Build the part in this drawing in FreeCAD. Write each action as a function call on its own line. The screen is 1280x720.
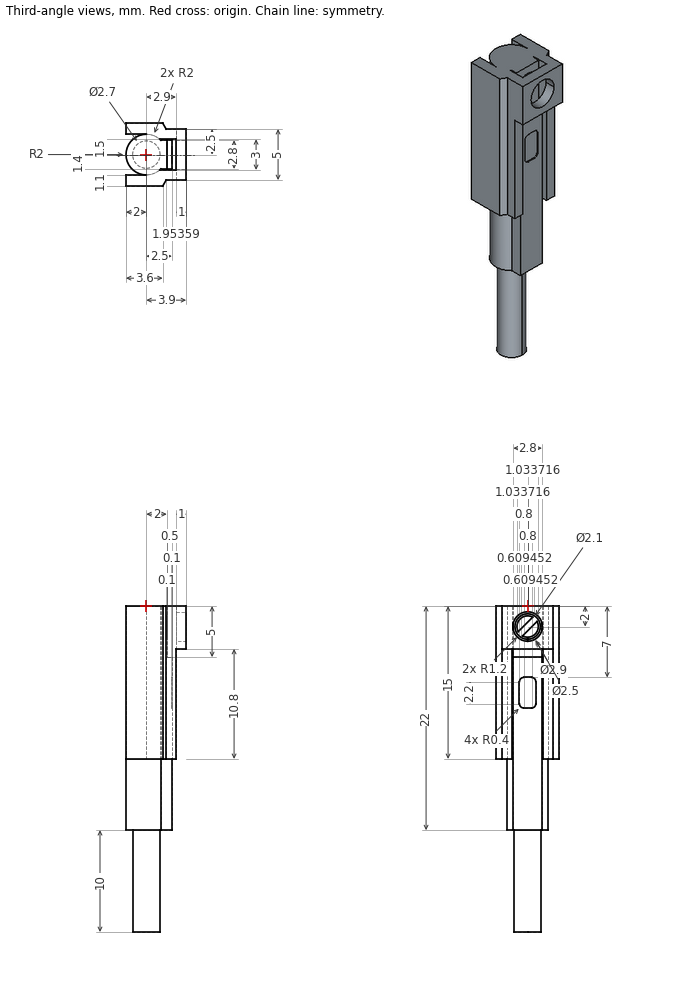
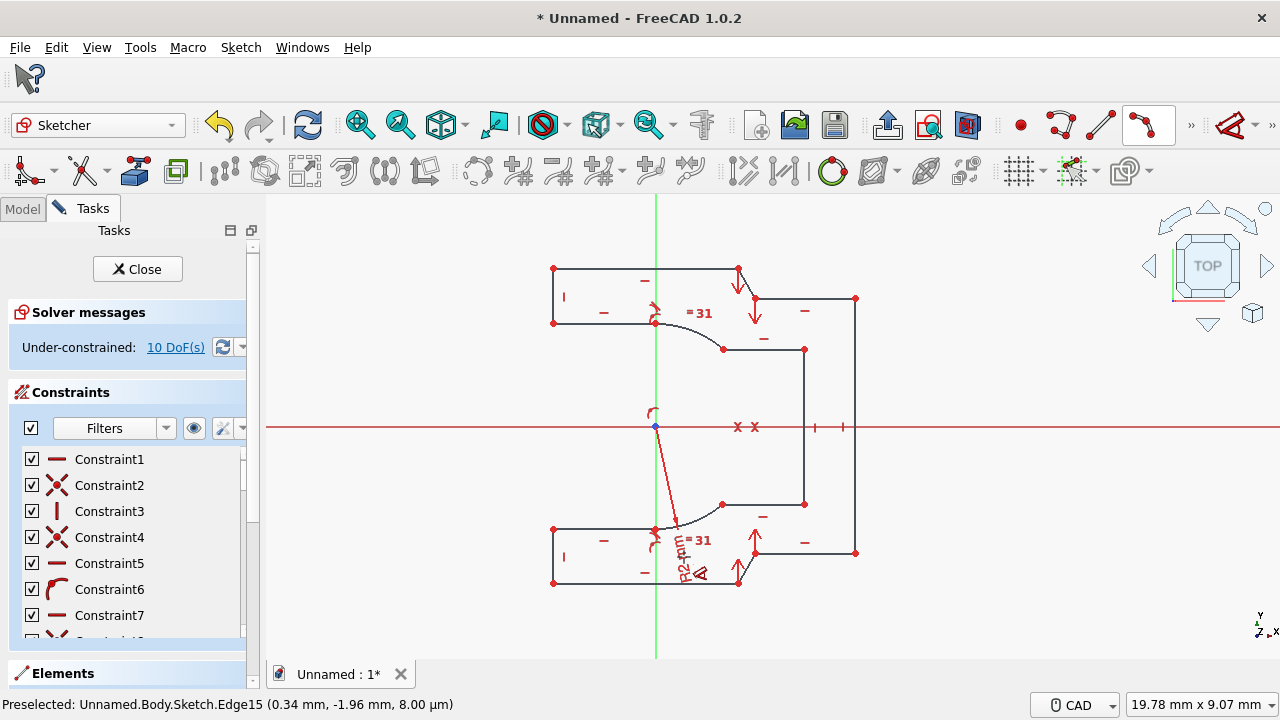
click(804, 396)
click(838, 392)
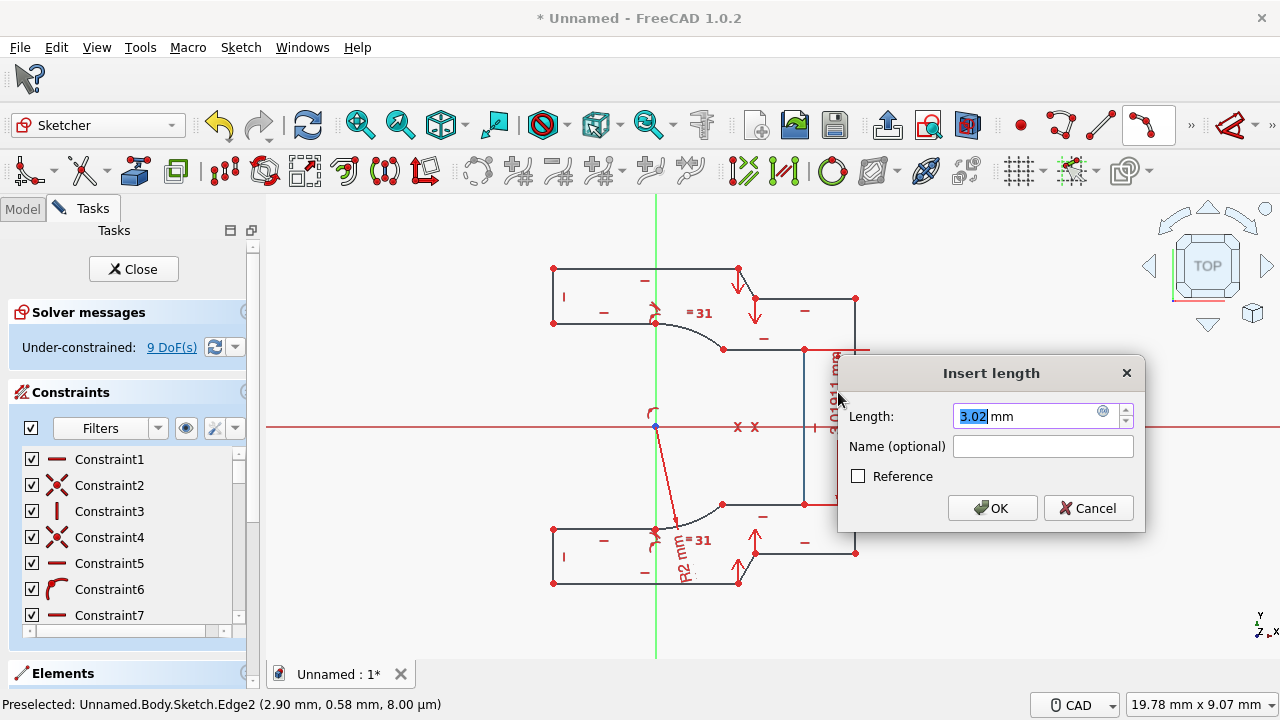
text(3)
key(Return)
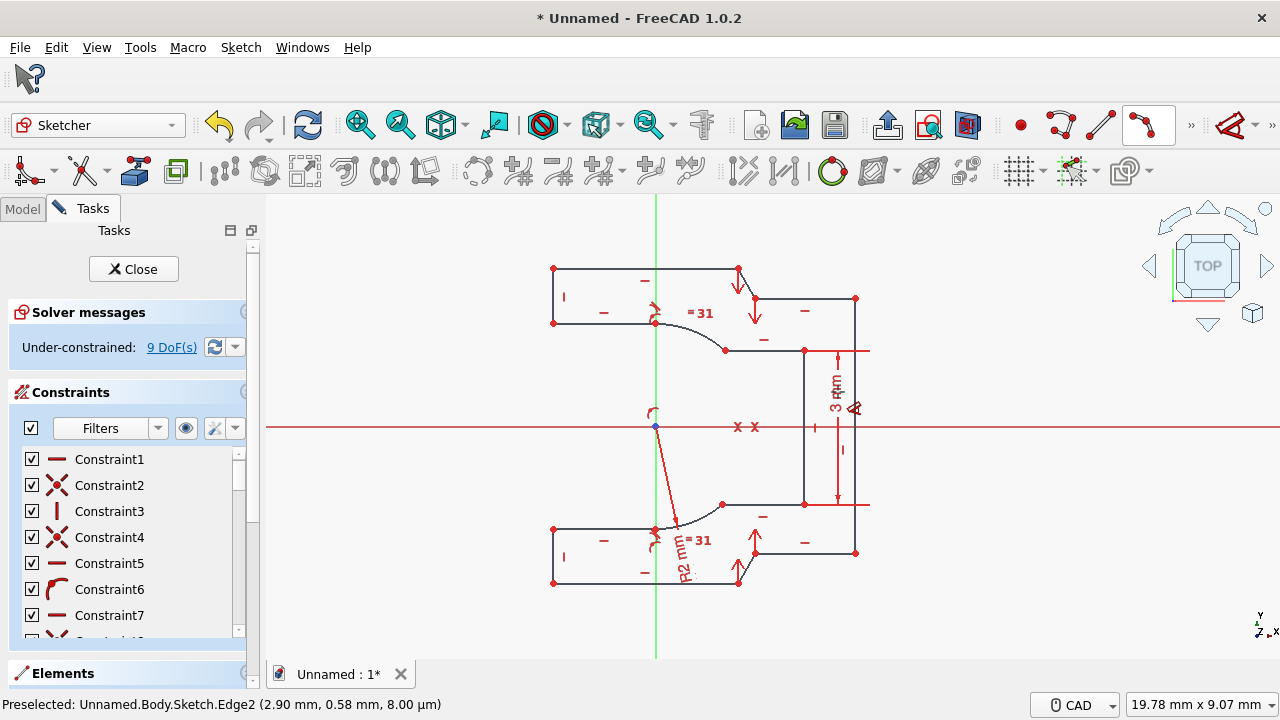
click(625, 529)
click(605, 563)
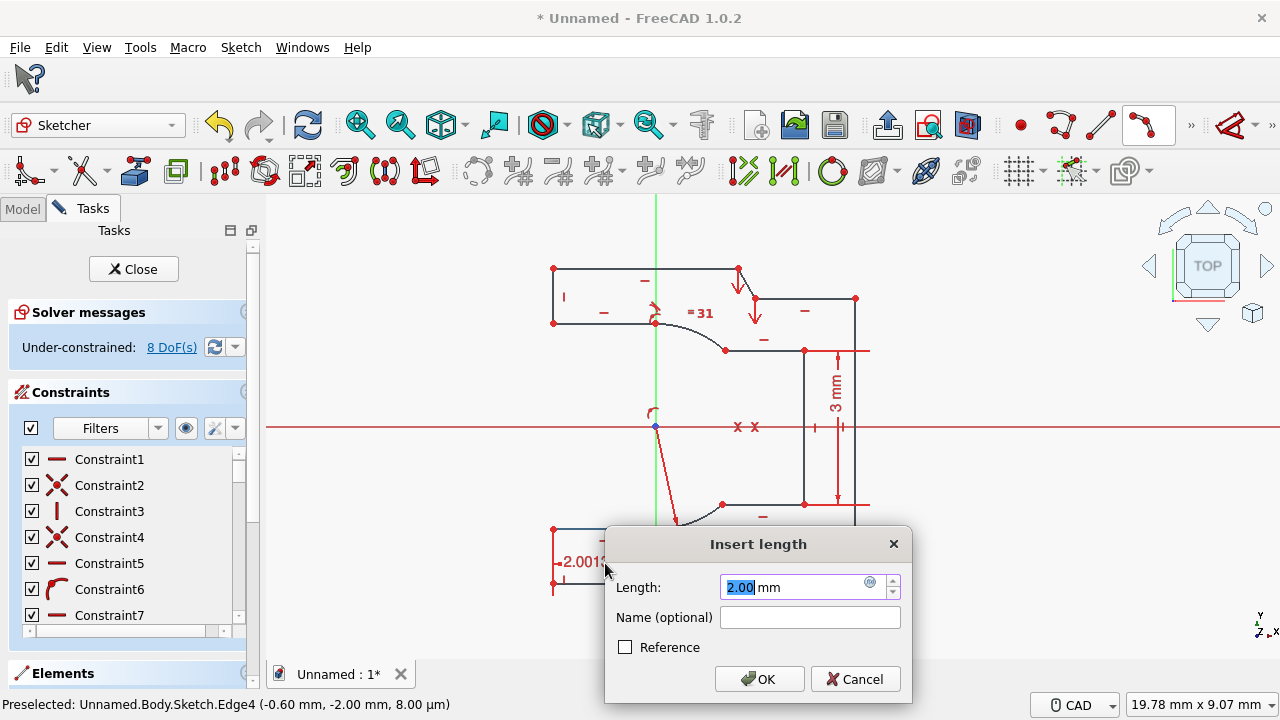
text(2)
key(Return)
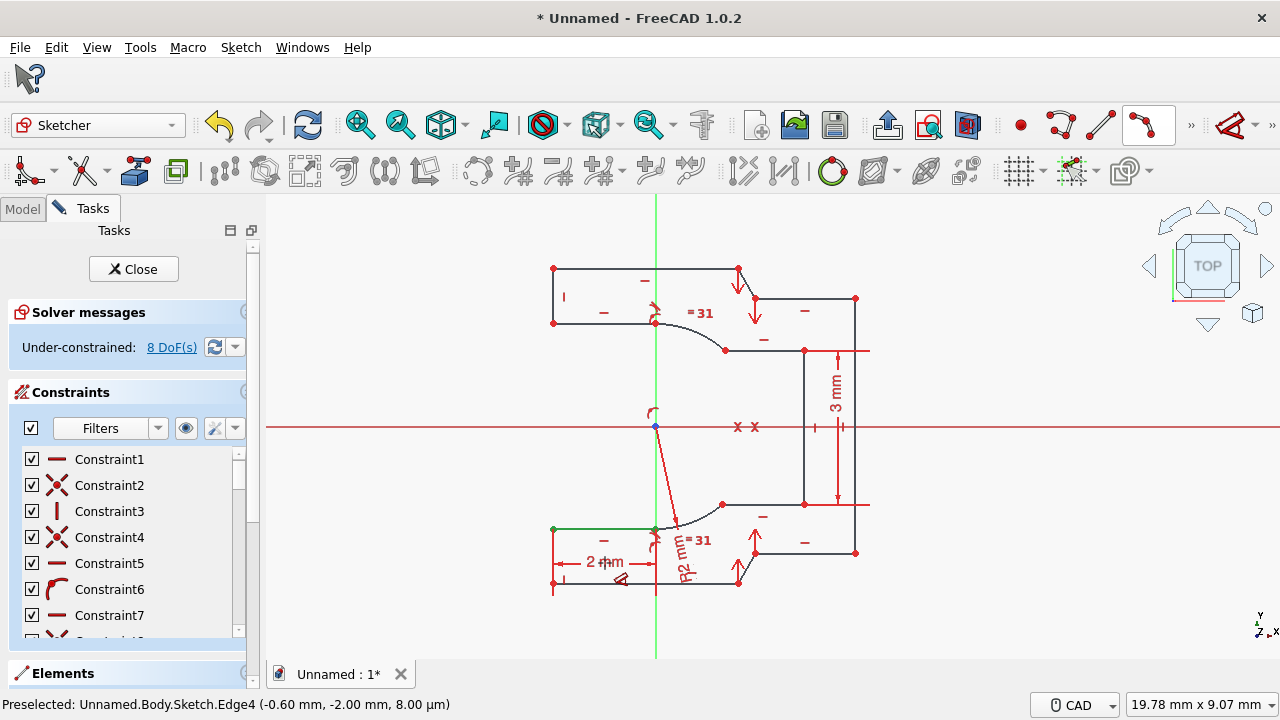
click(855, 477)
click(889, 368)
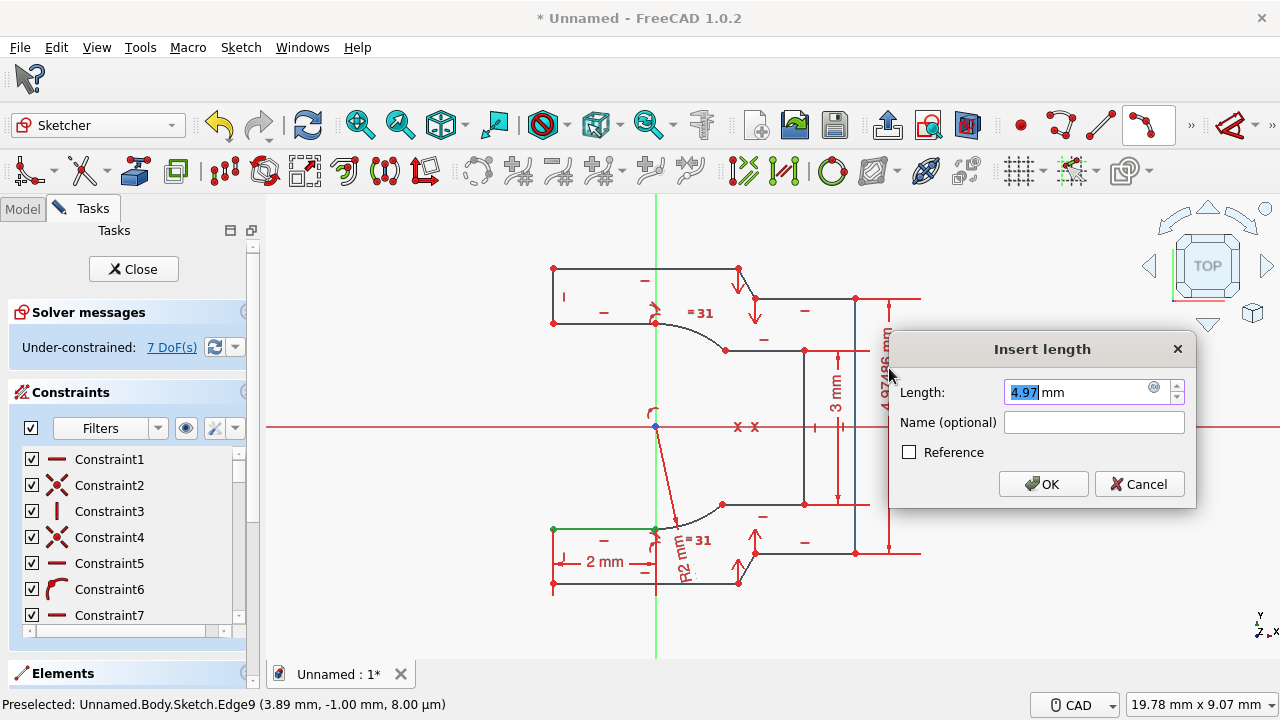
text(5)
key(Return)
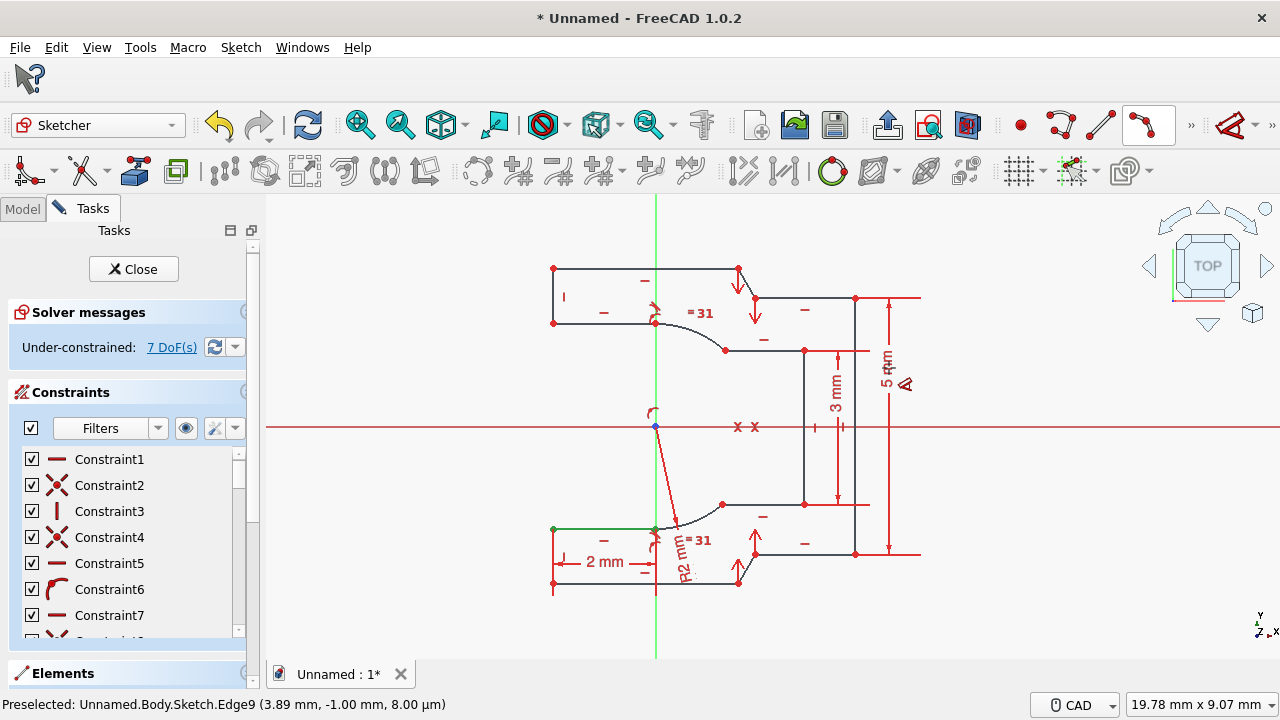
click(584, 324)
click(605, 290)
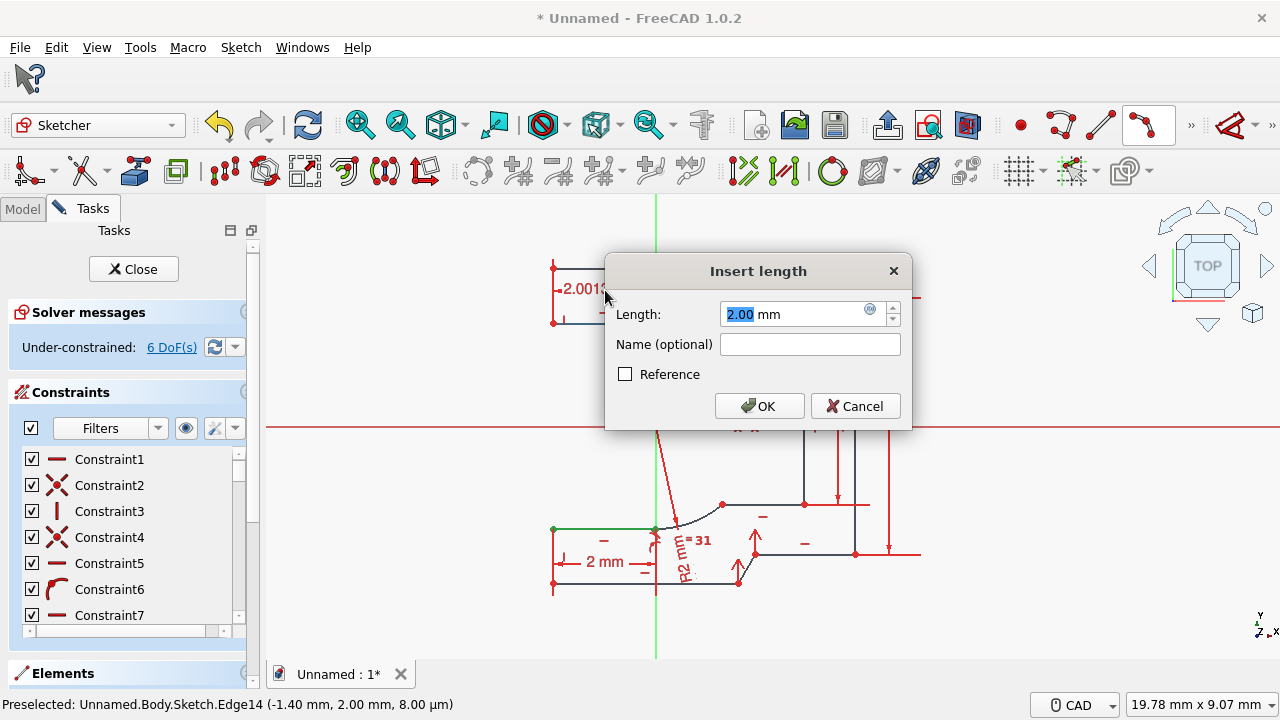
text(2)
key(Return)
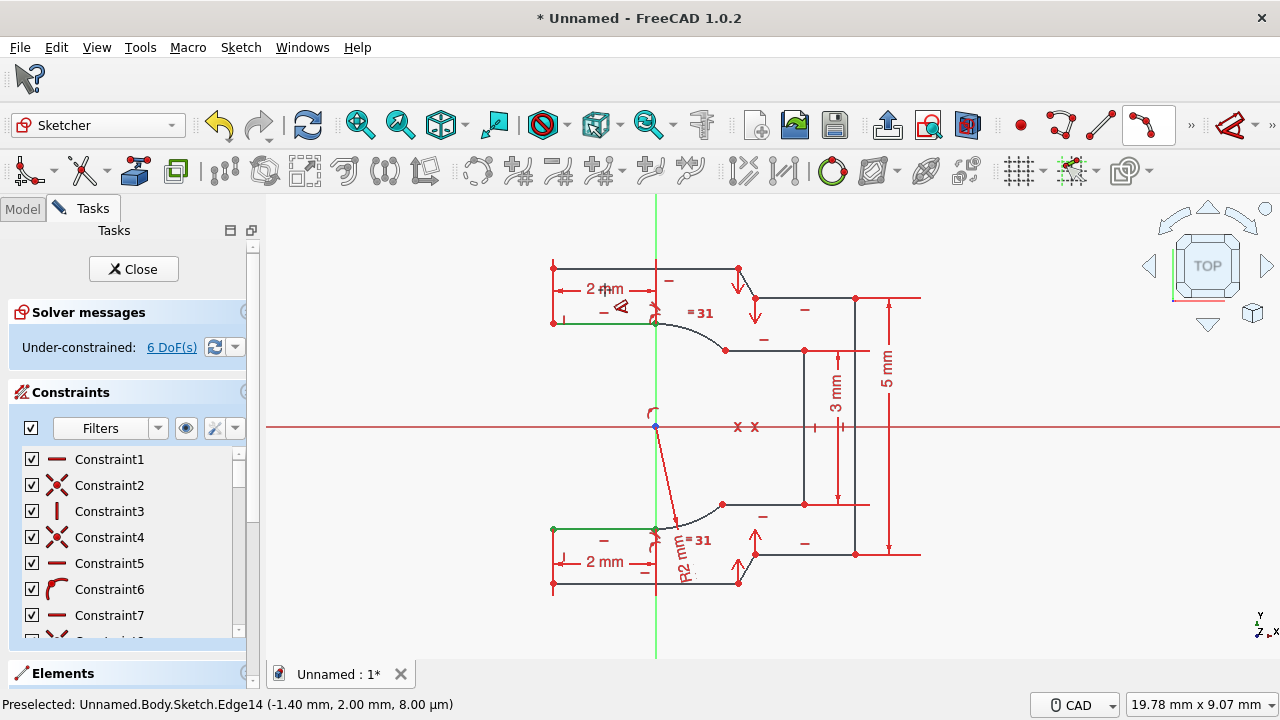
click(553, 546)
click(519, 557)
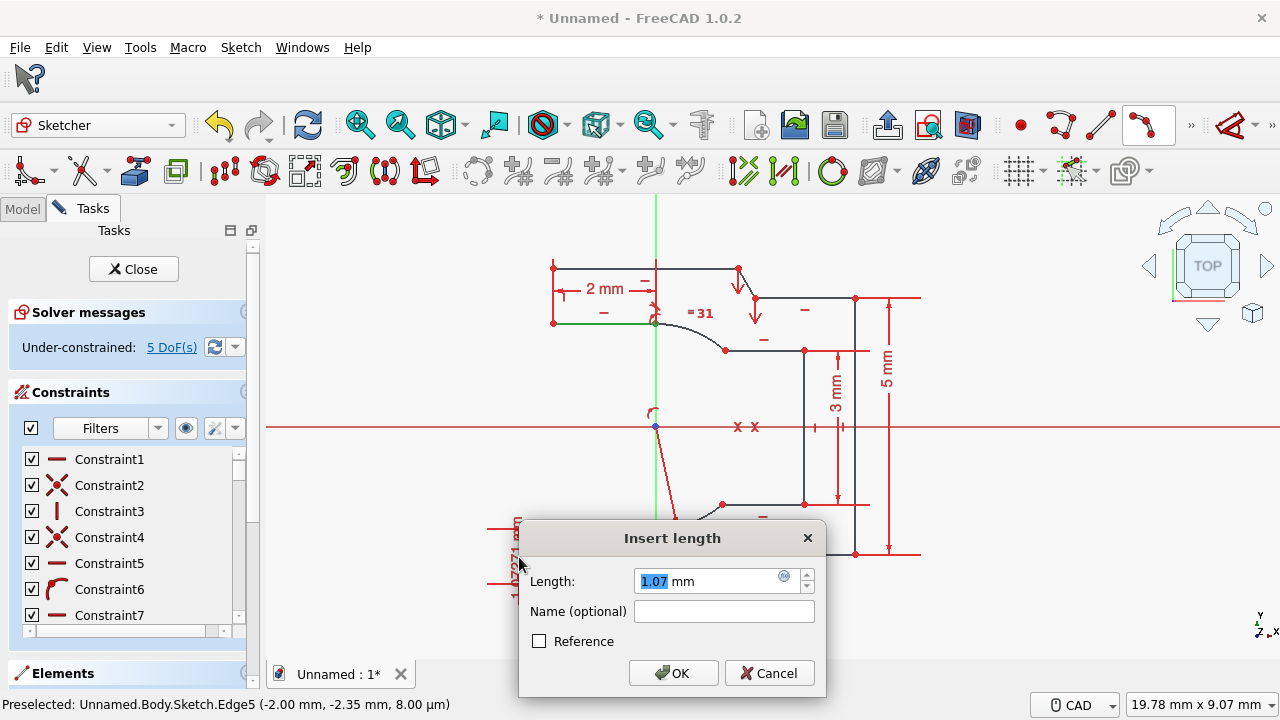
text(1.1)
key(Return)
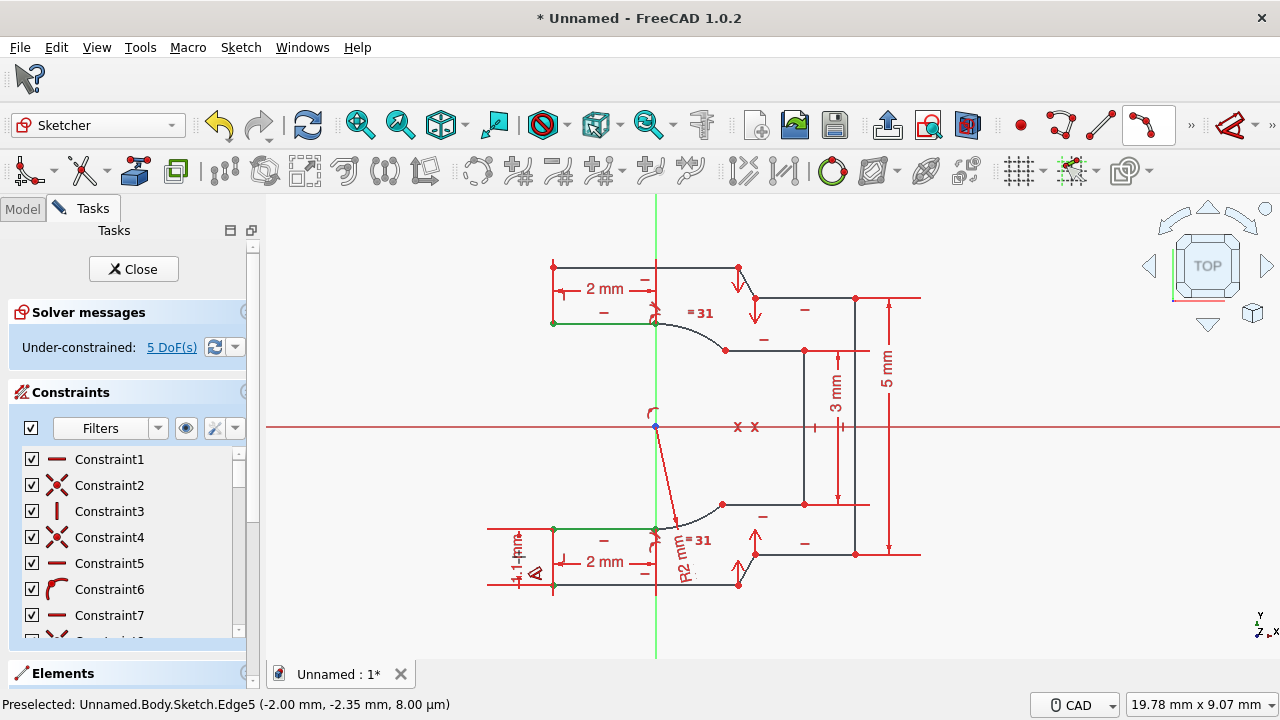
click(609, 585)
click(603, 619)